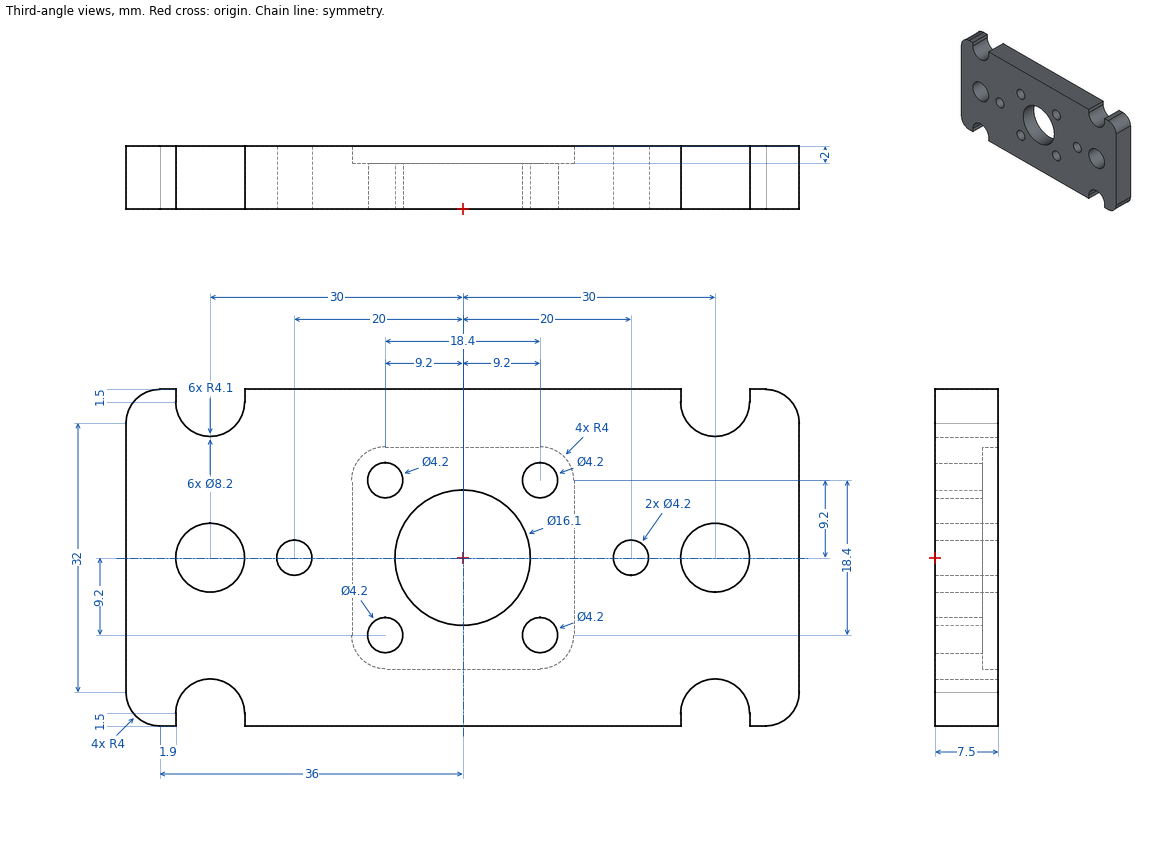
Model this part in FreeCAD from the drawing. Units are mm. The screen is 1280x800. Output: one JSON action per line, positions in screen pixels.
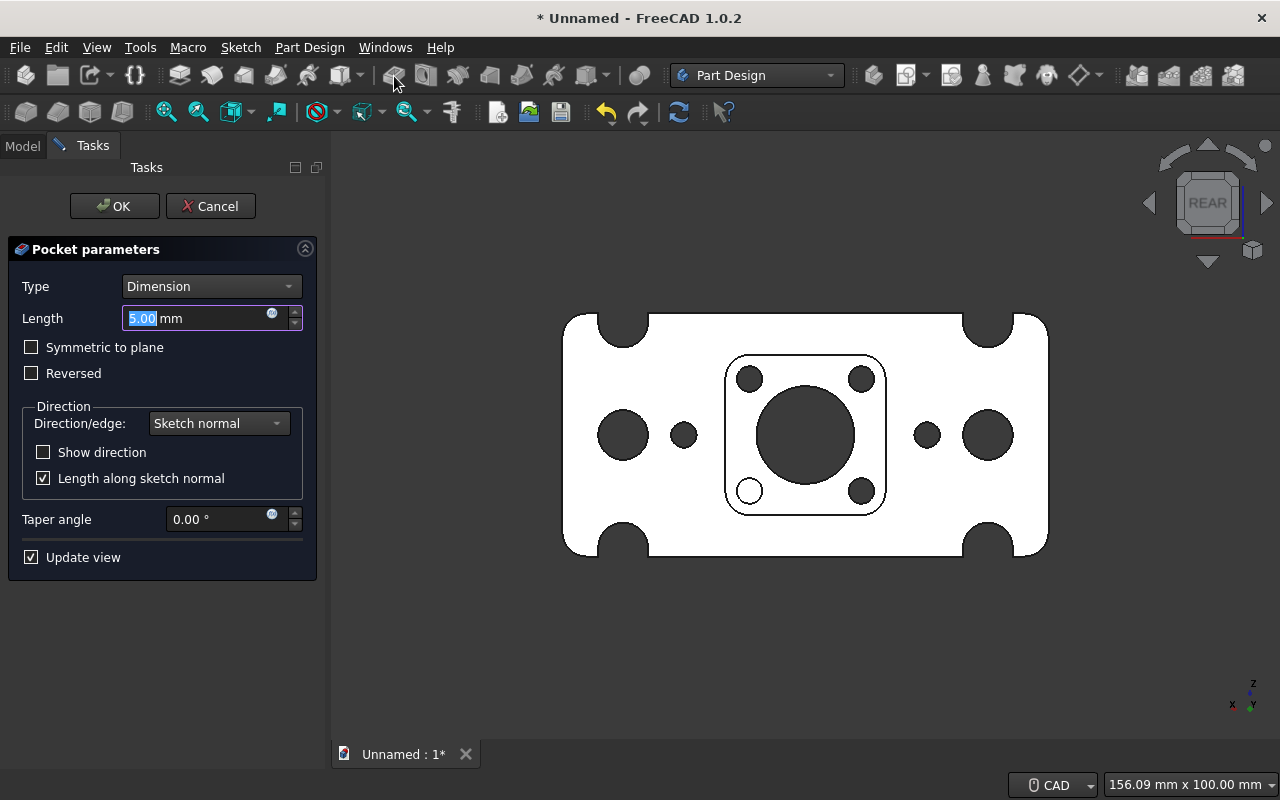
{"action": "left_click", "coordinate": [212, 286]}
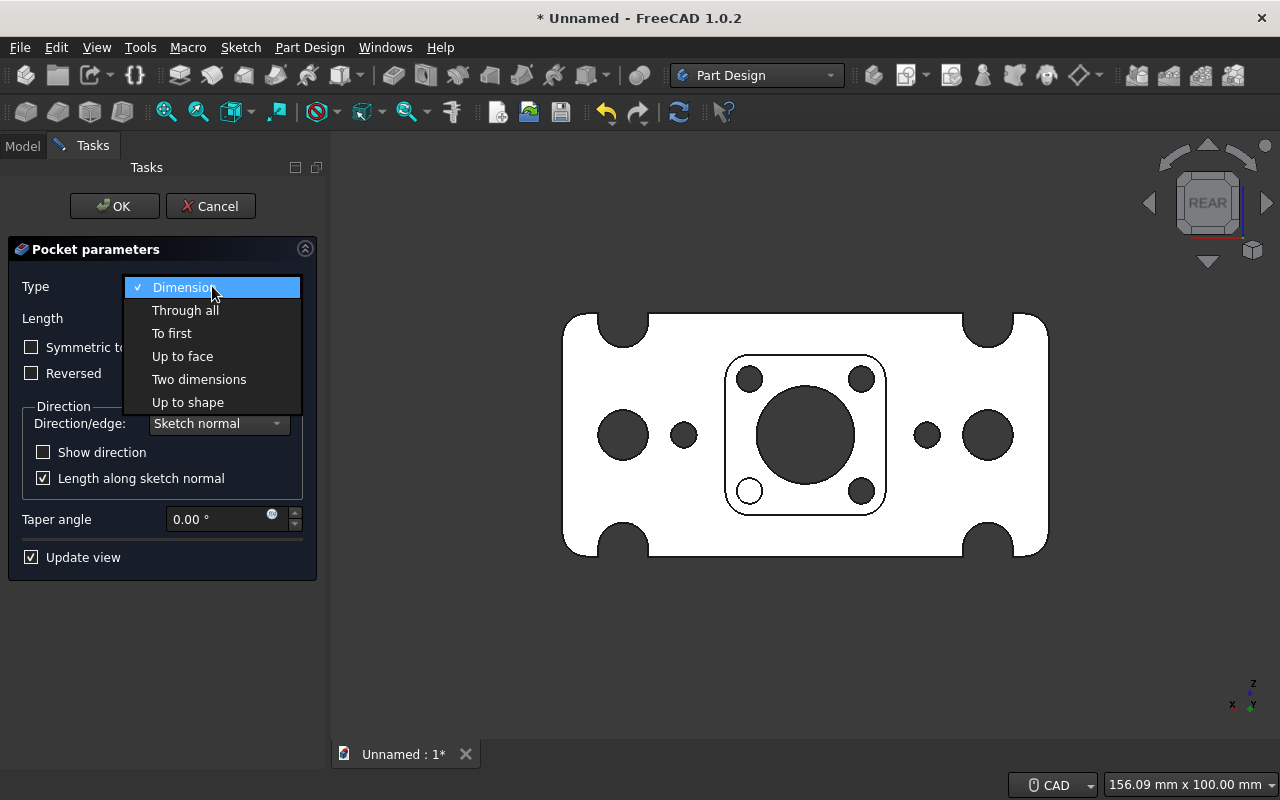
{"action": "left_click", "coordinate": [212, 334]}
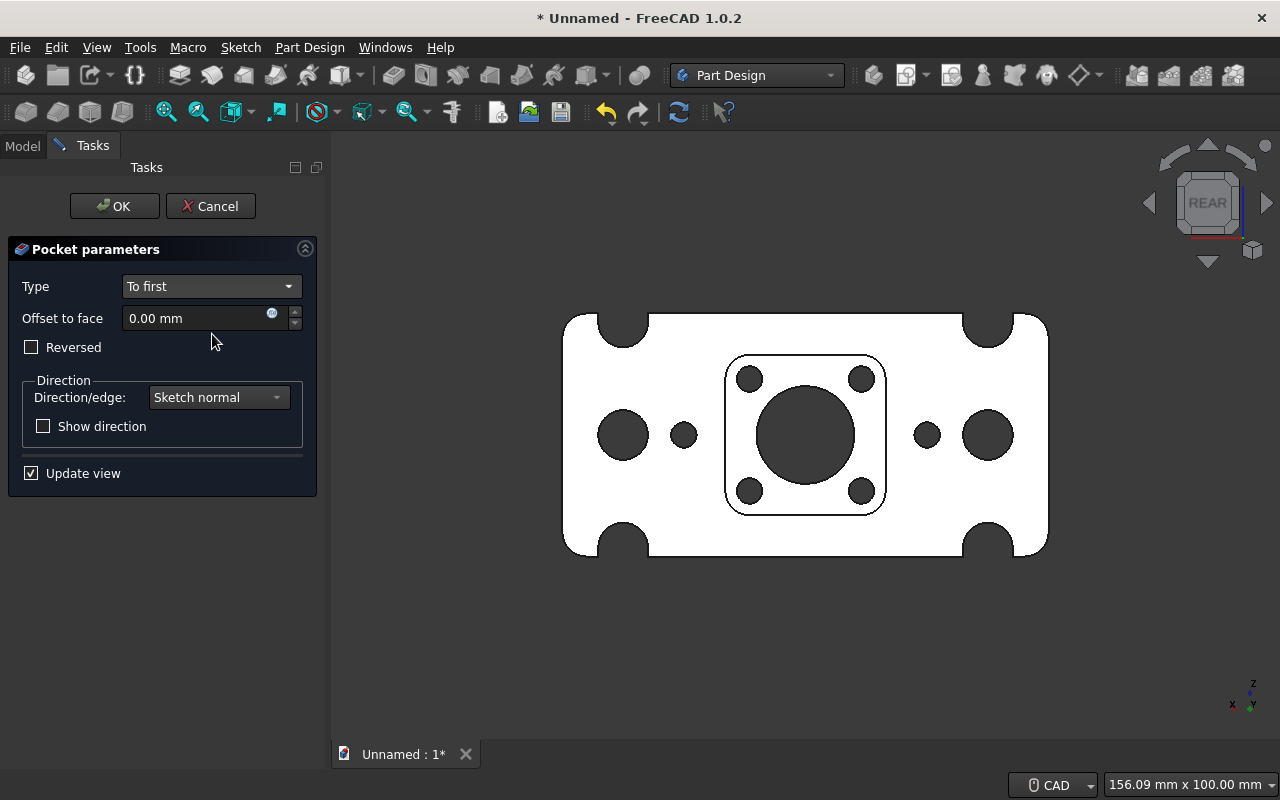
{"action": "left_click", "coordinate": [115, 206]}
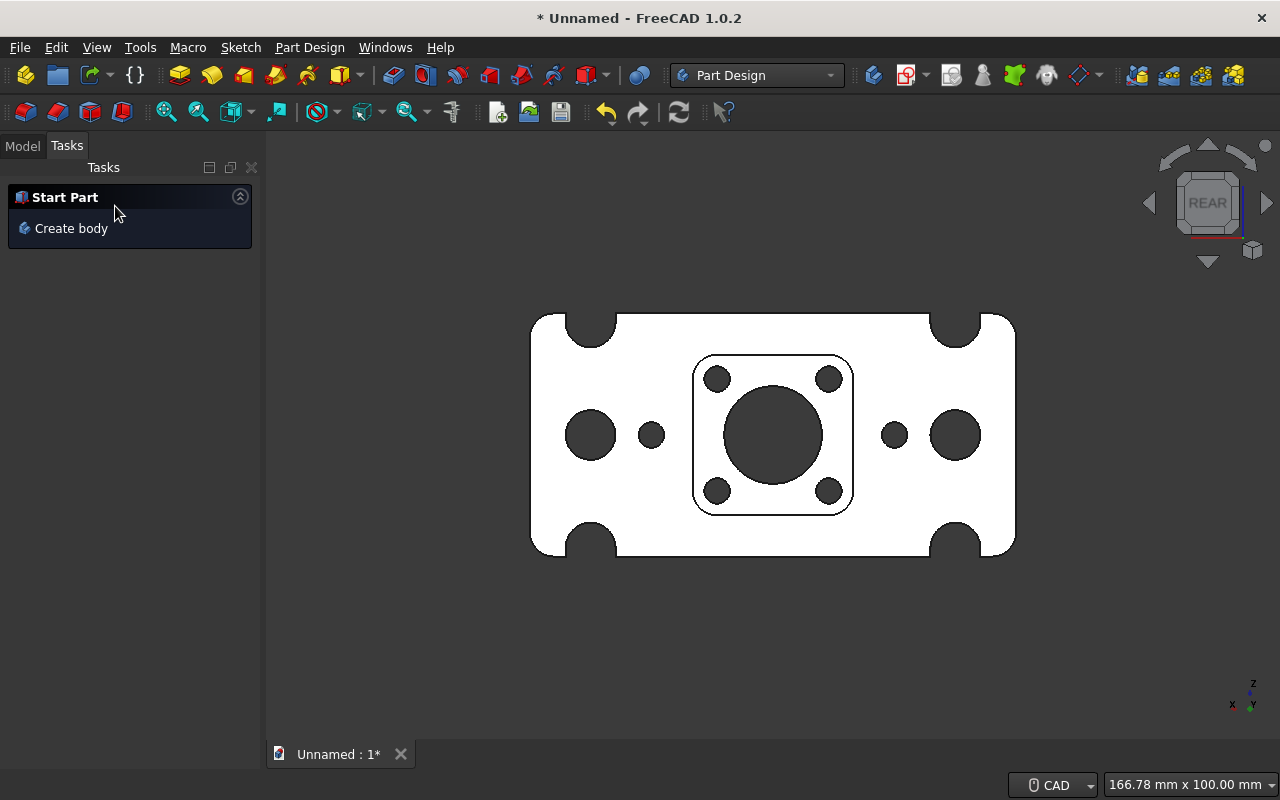
{"action": "key", "text": "0"}